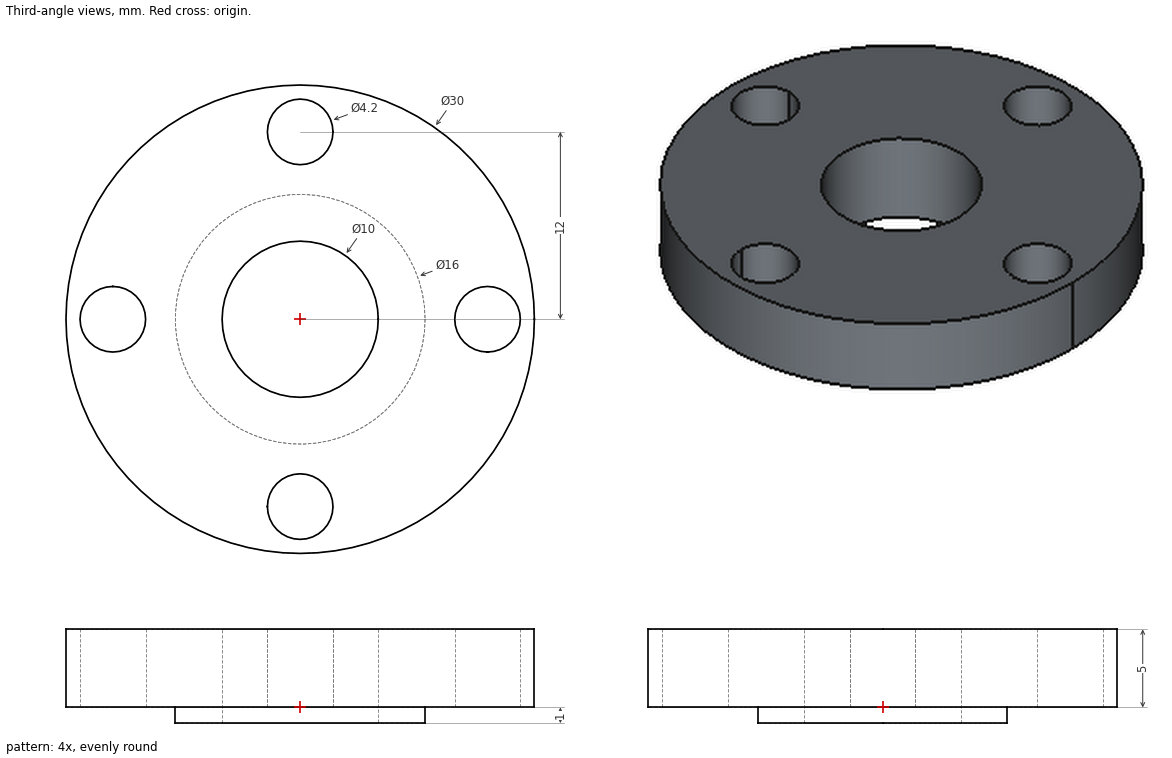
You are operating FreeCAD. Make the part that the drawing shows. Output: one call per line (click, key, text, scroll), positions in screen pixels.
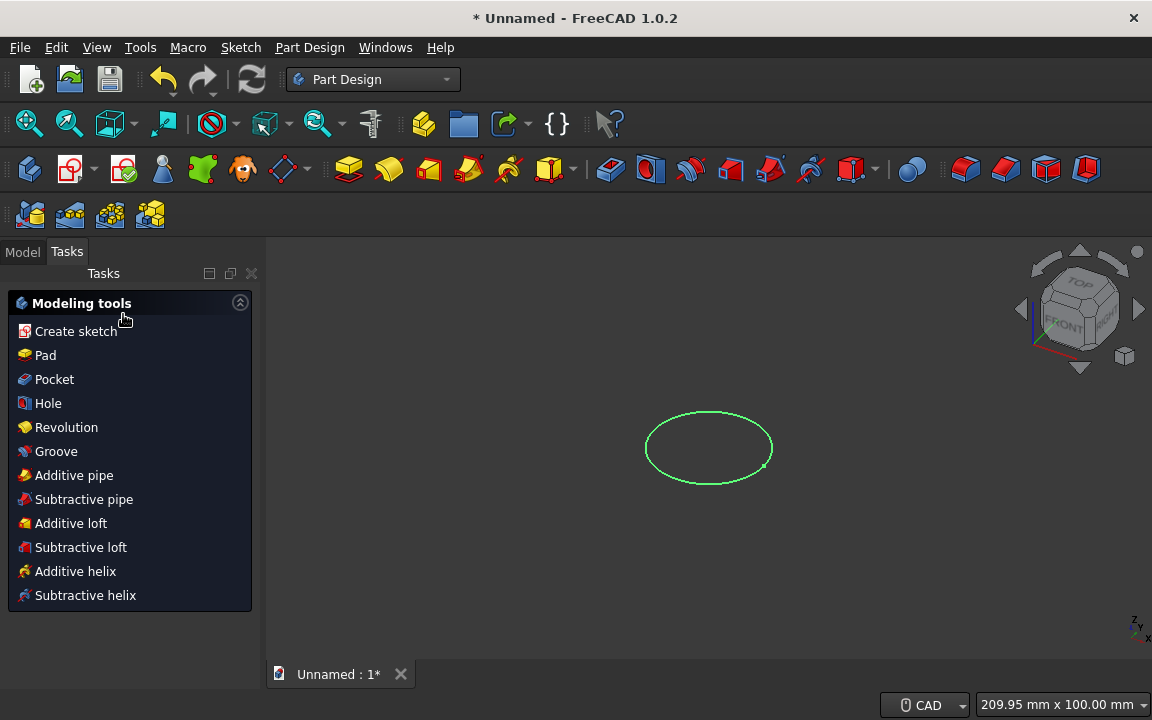
click(350, 170)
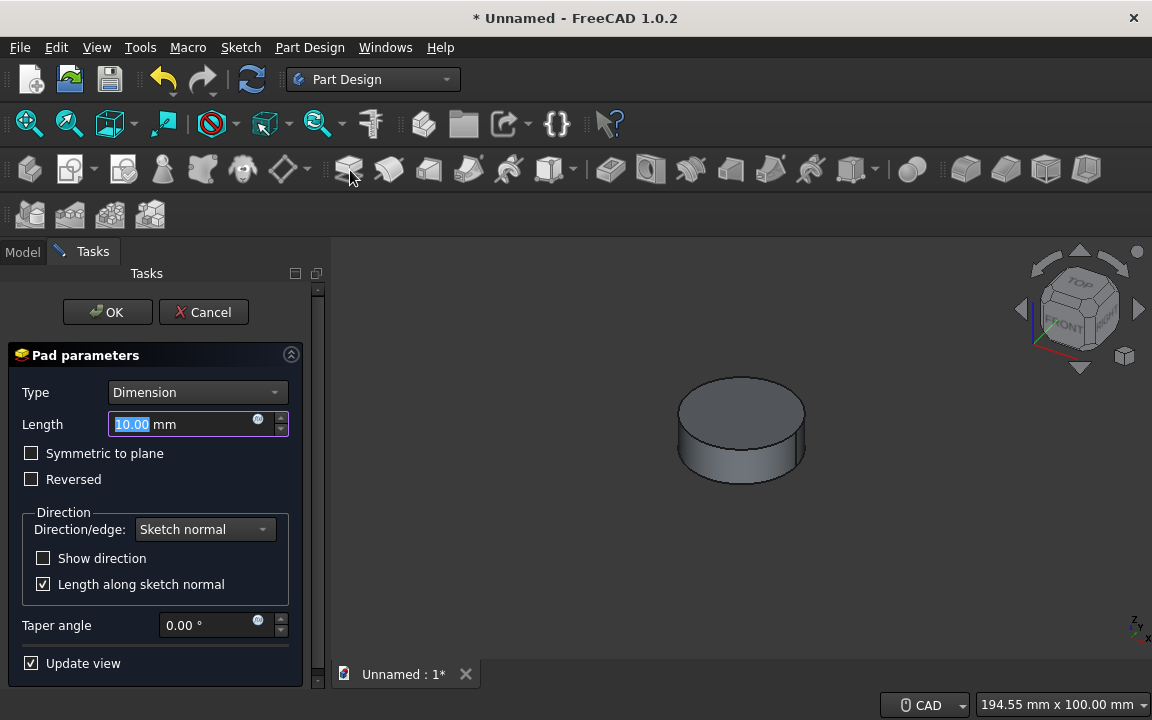
text(5)
key(Tab)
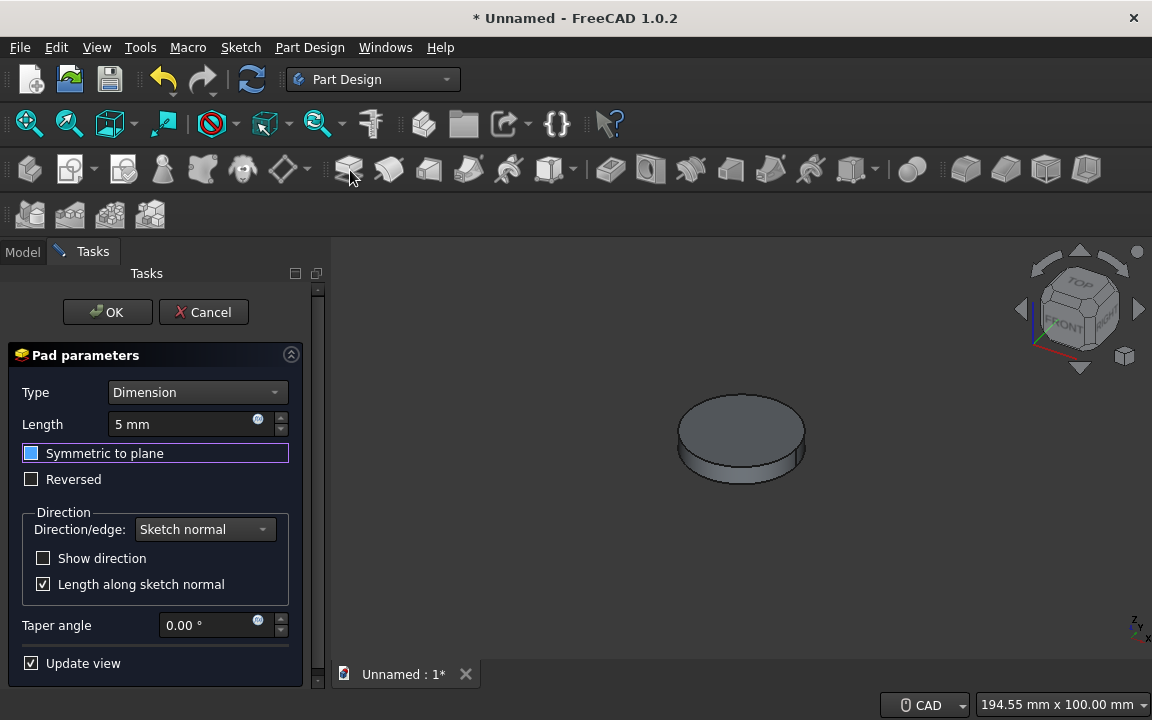
click(108, 312)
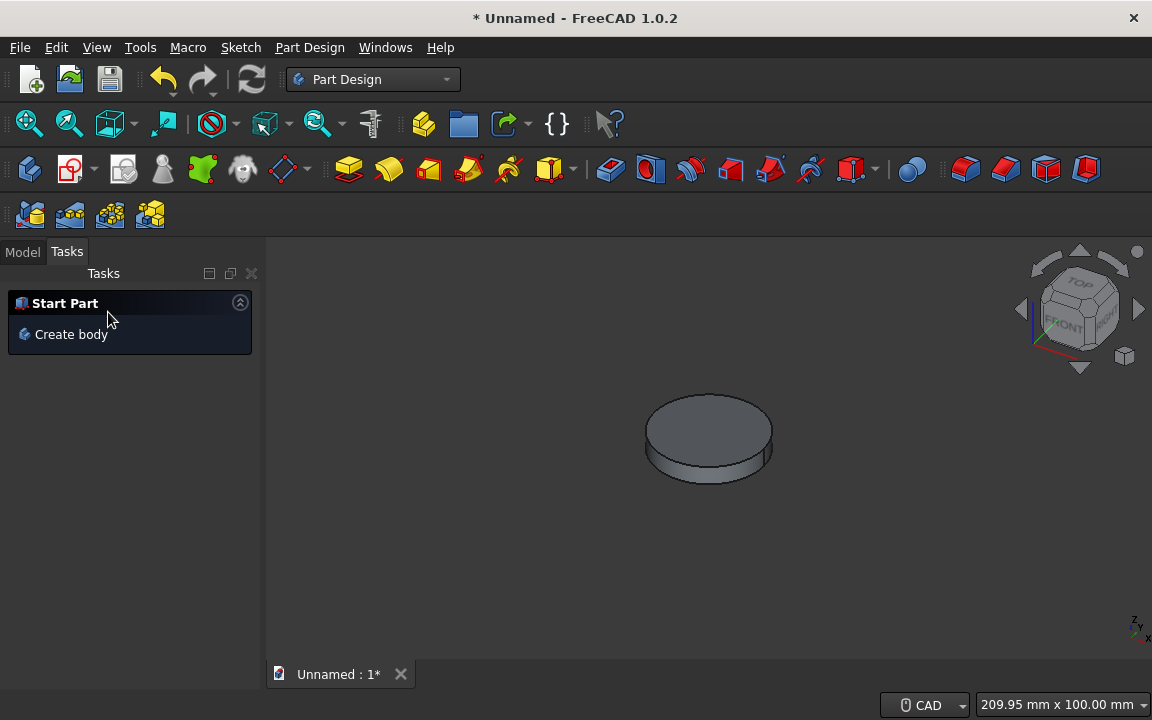
click(30, 124)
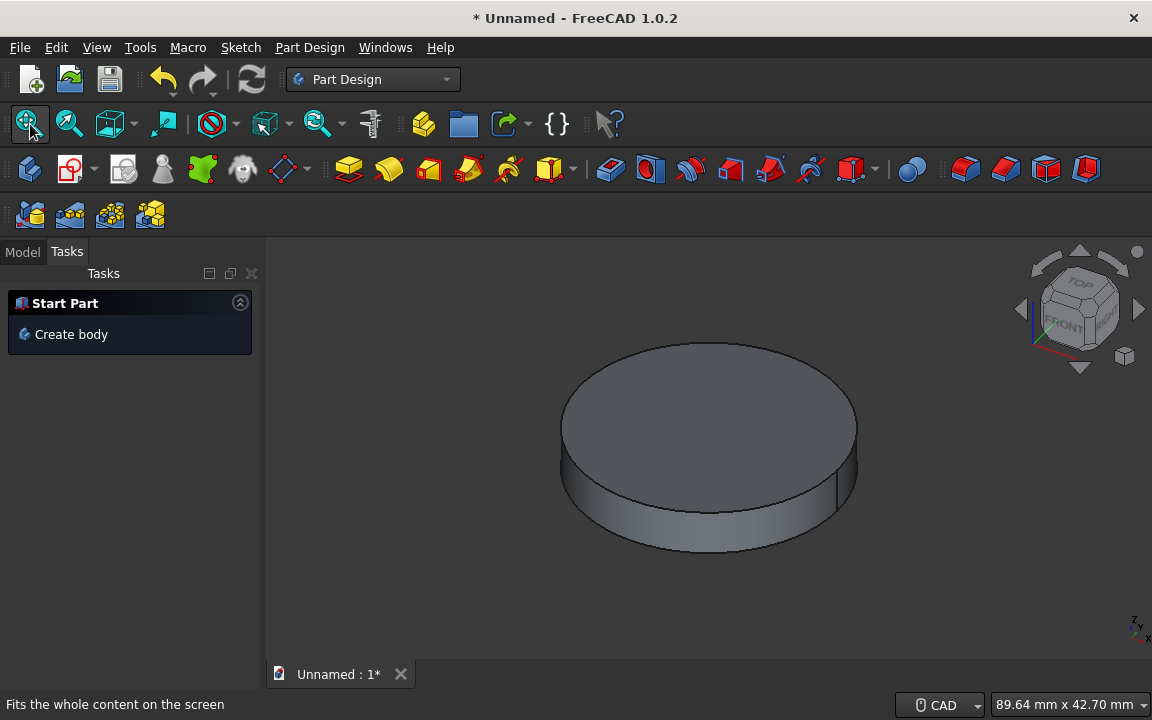
click(709, 427)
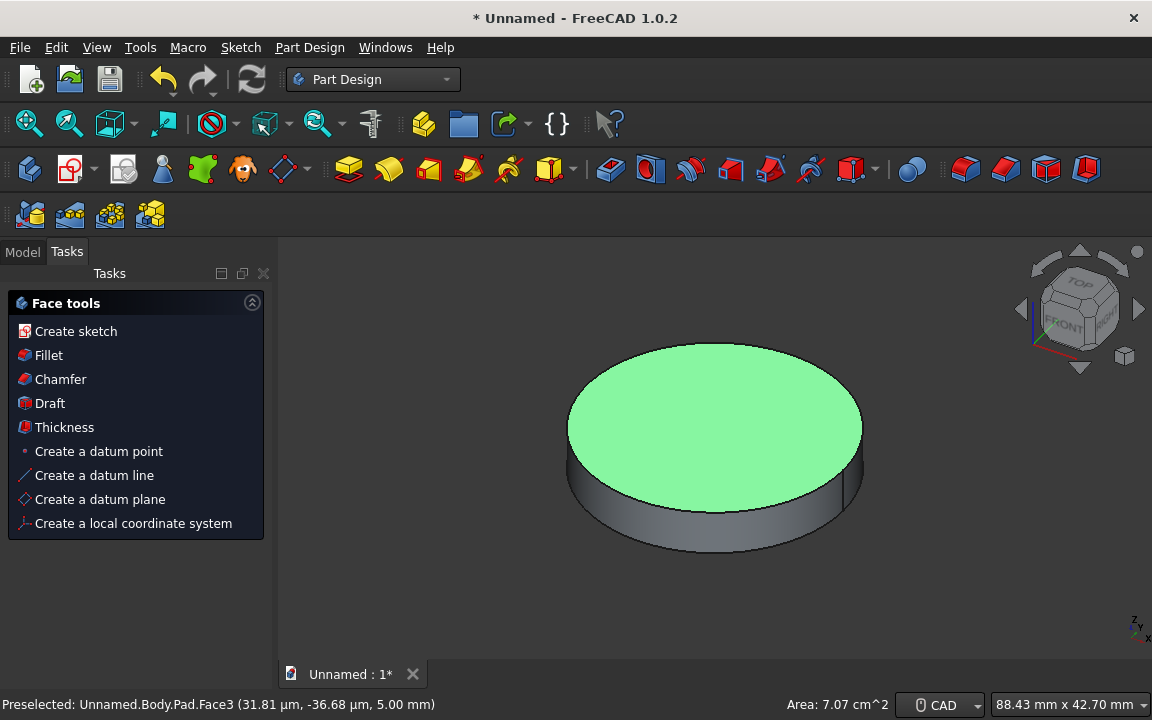
click(70, 170)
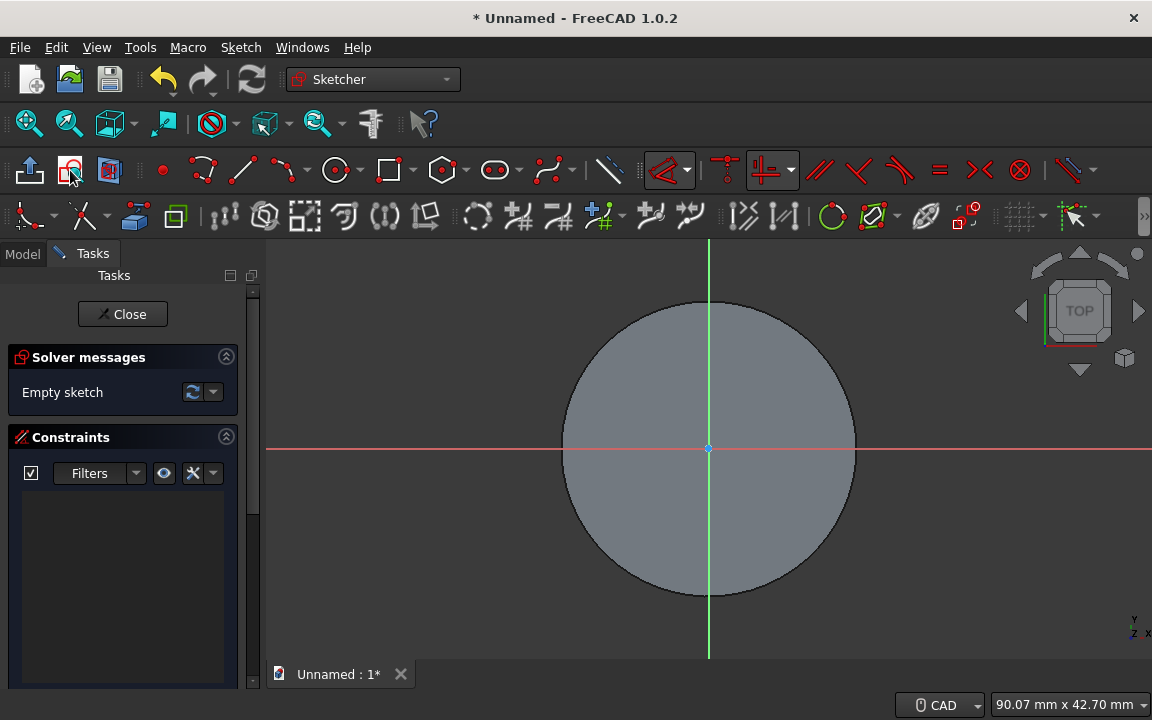
scroll(722, 308, up, 9)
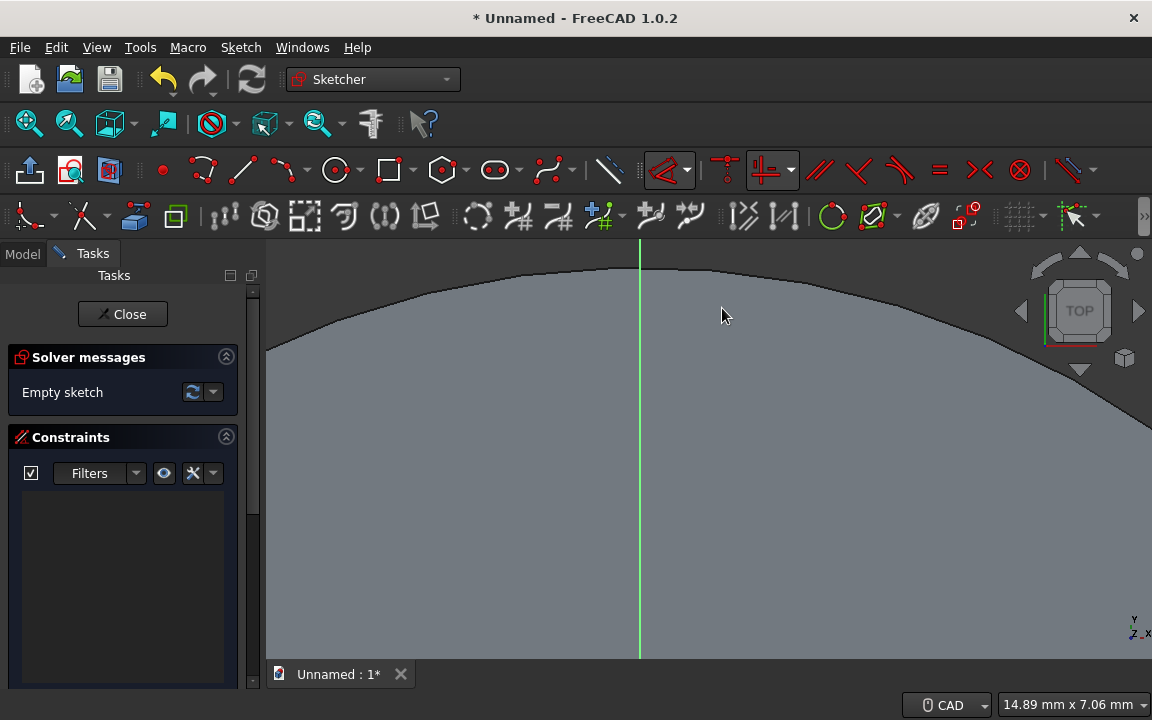
key(g)
key(c)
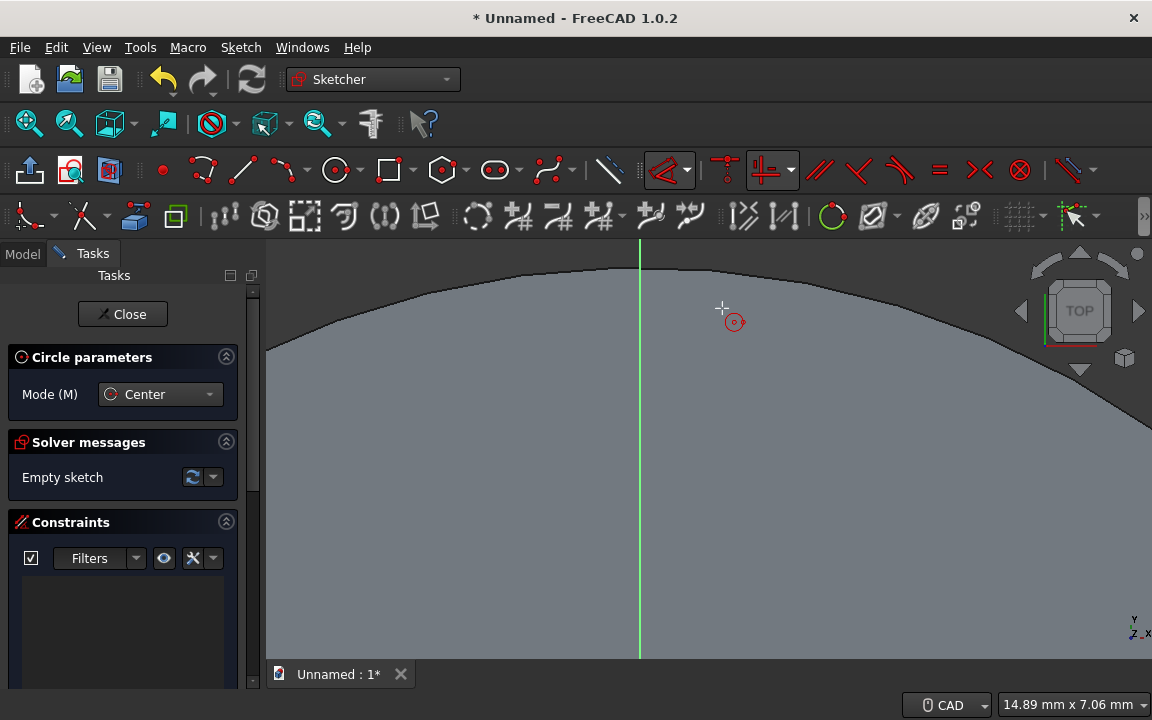
click(640, 446)
click(728, 358)
key(Escape)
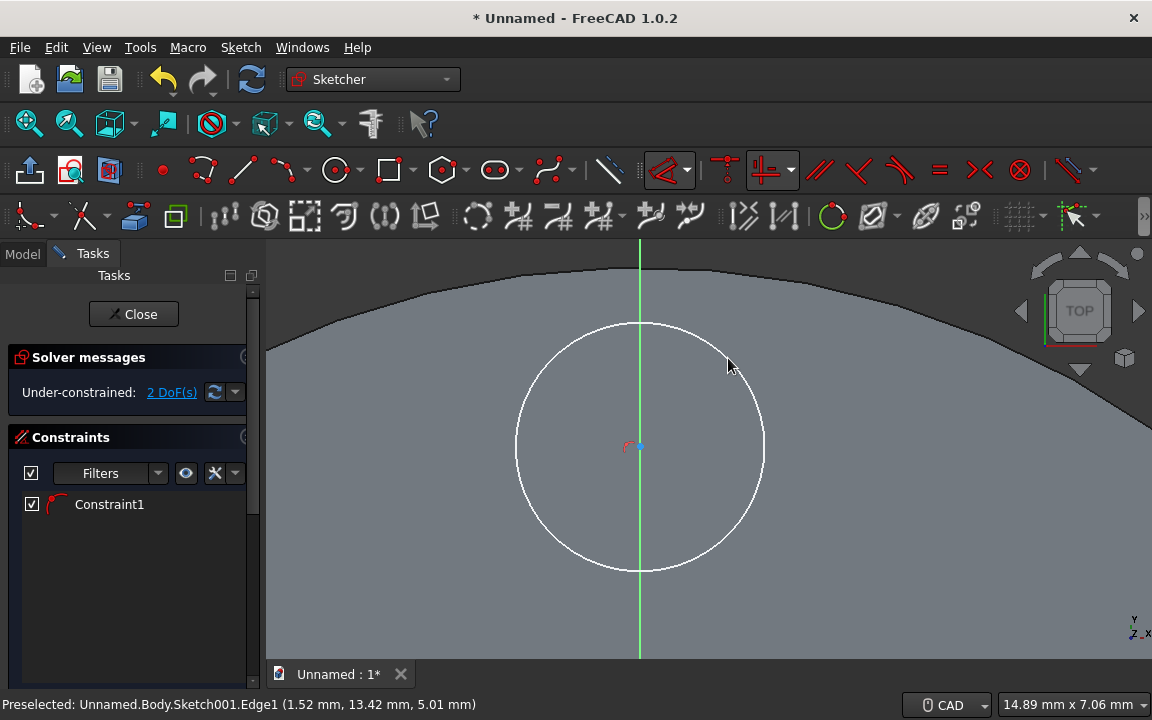
click(728, 359)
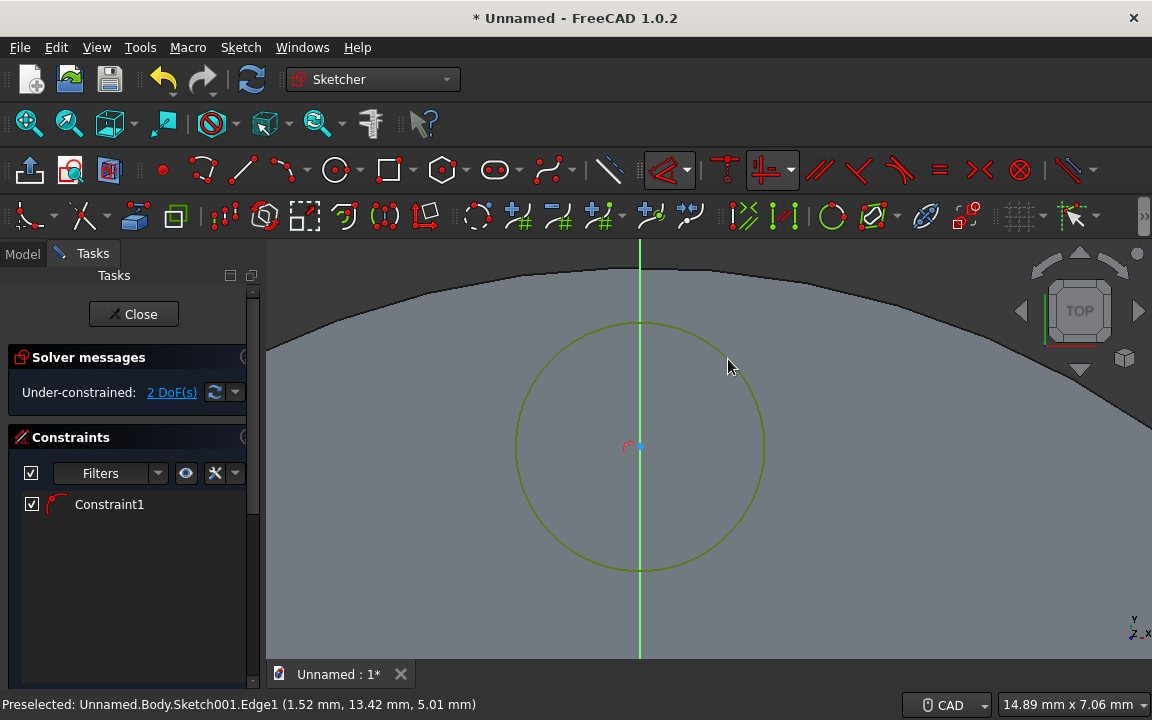
click(690, 170)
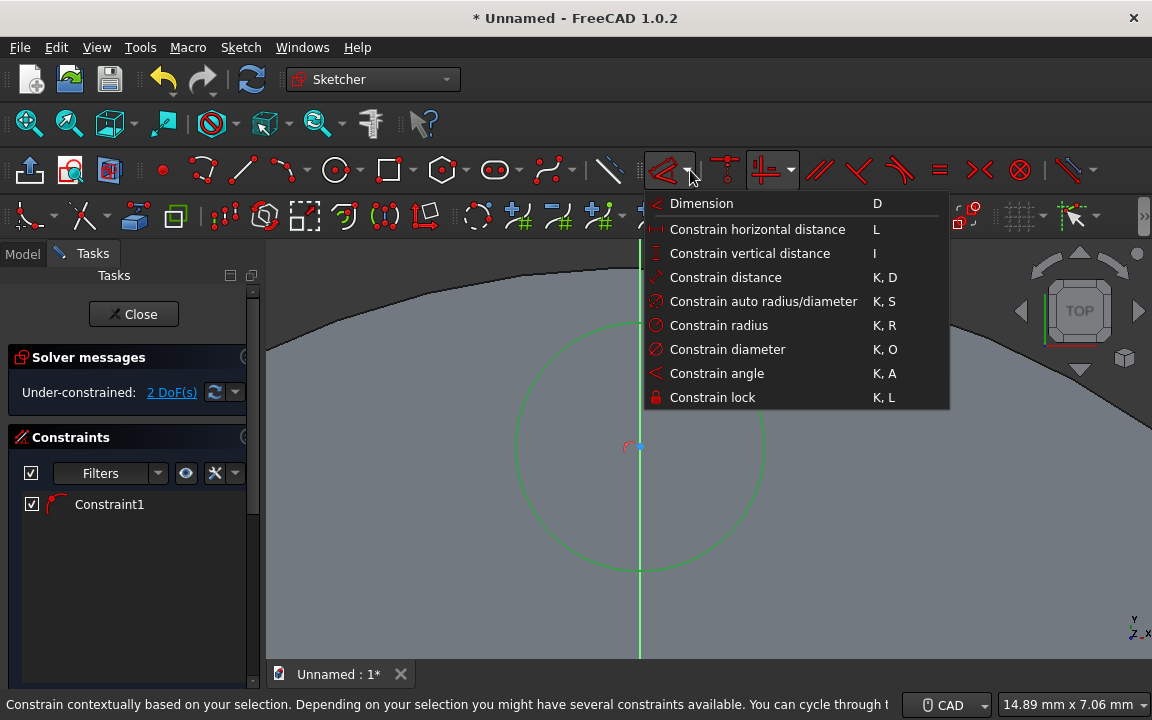
click(797, 349)